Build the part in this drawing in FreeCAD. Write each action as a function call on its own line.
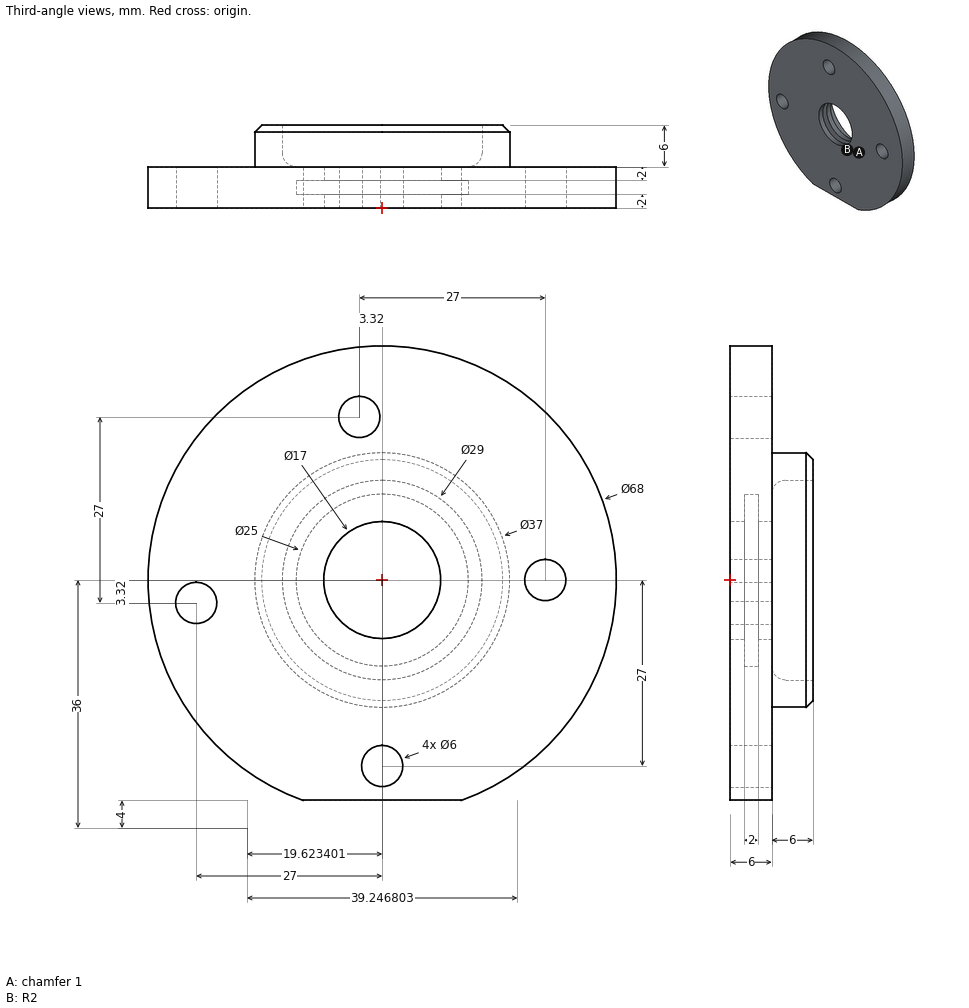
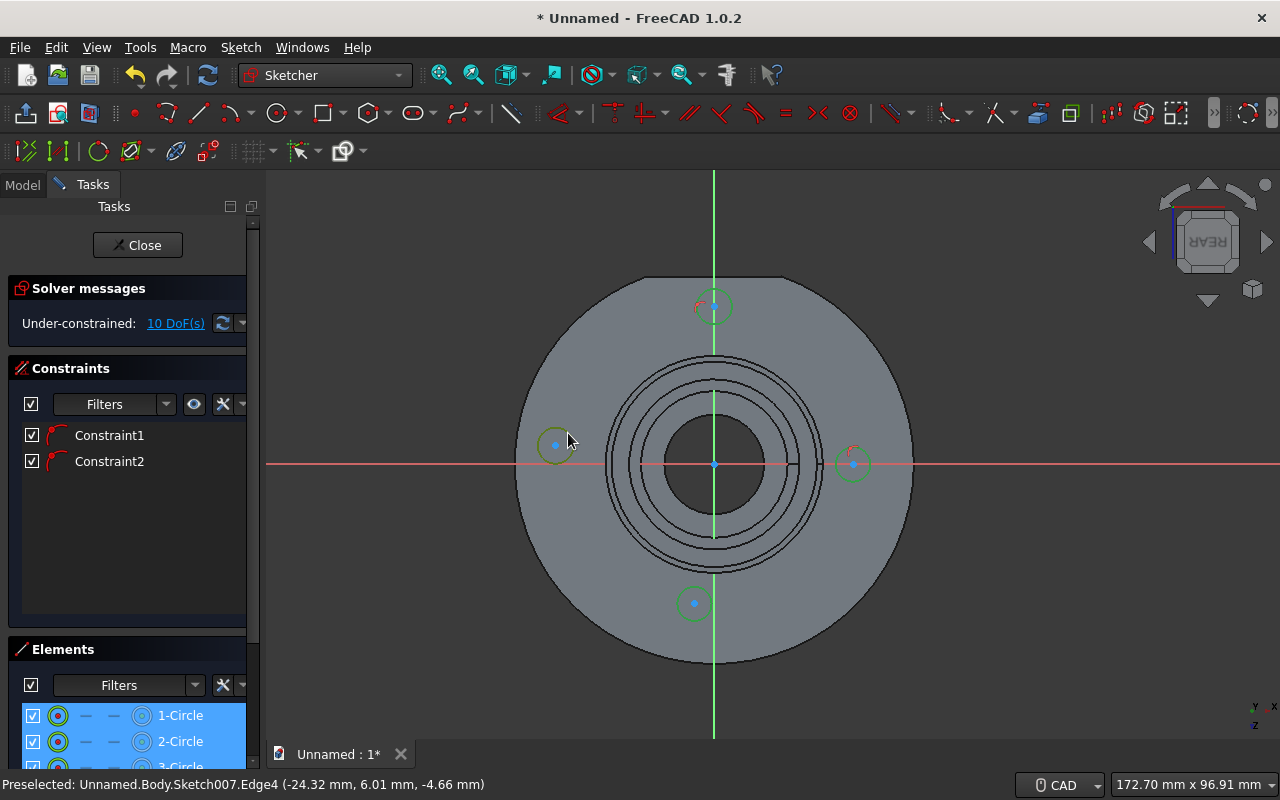
click(786, 114)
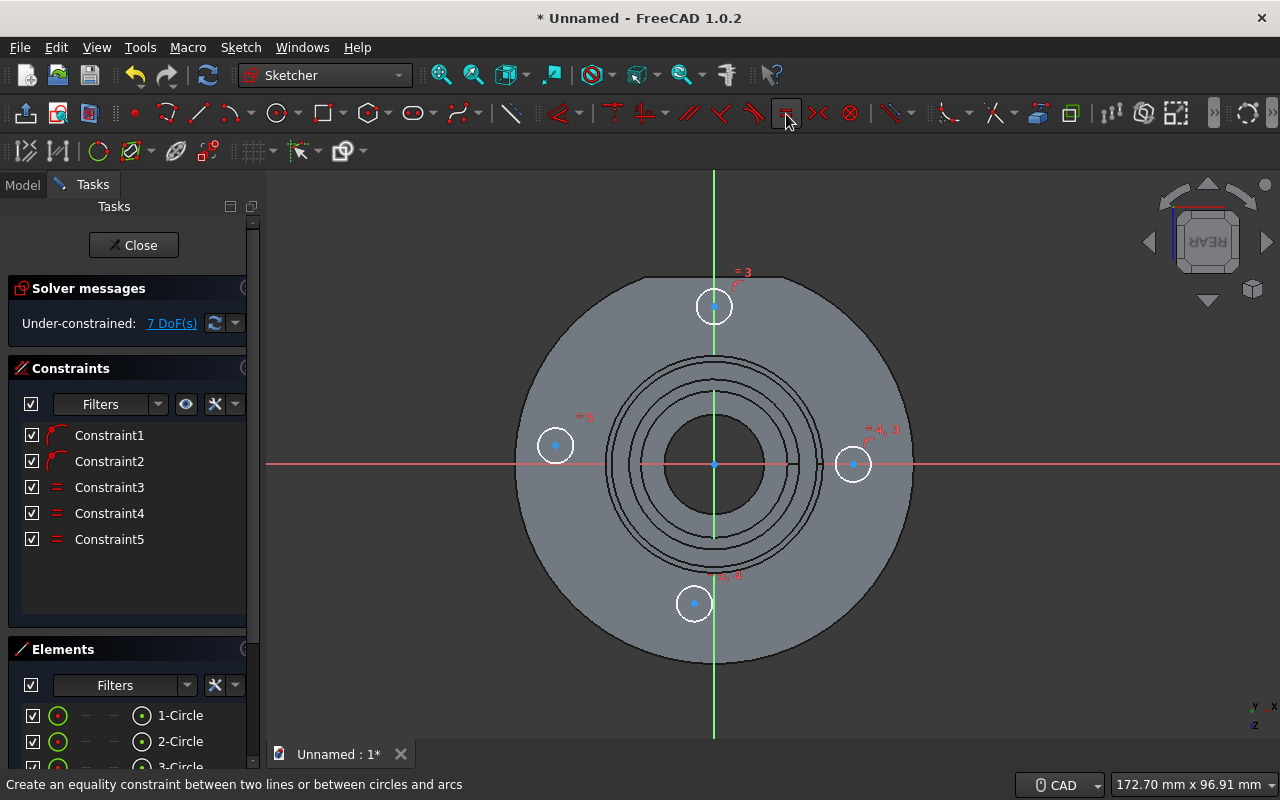
click(558, 114)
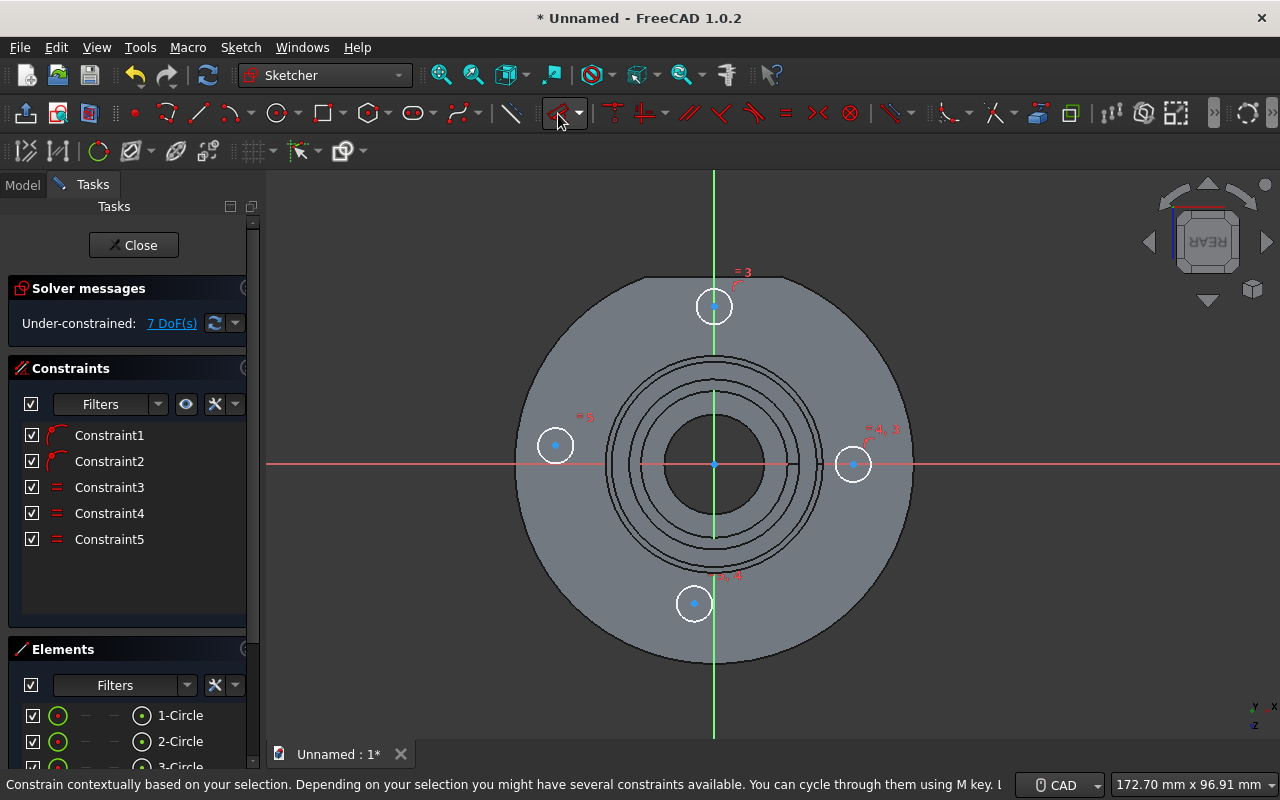
click(727, 294)
click(750, 271)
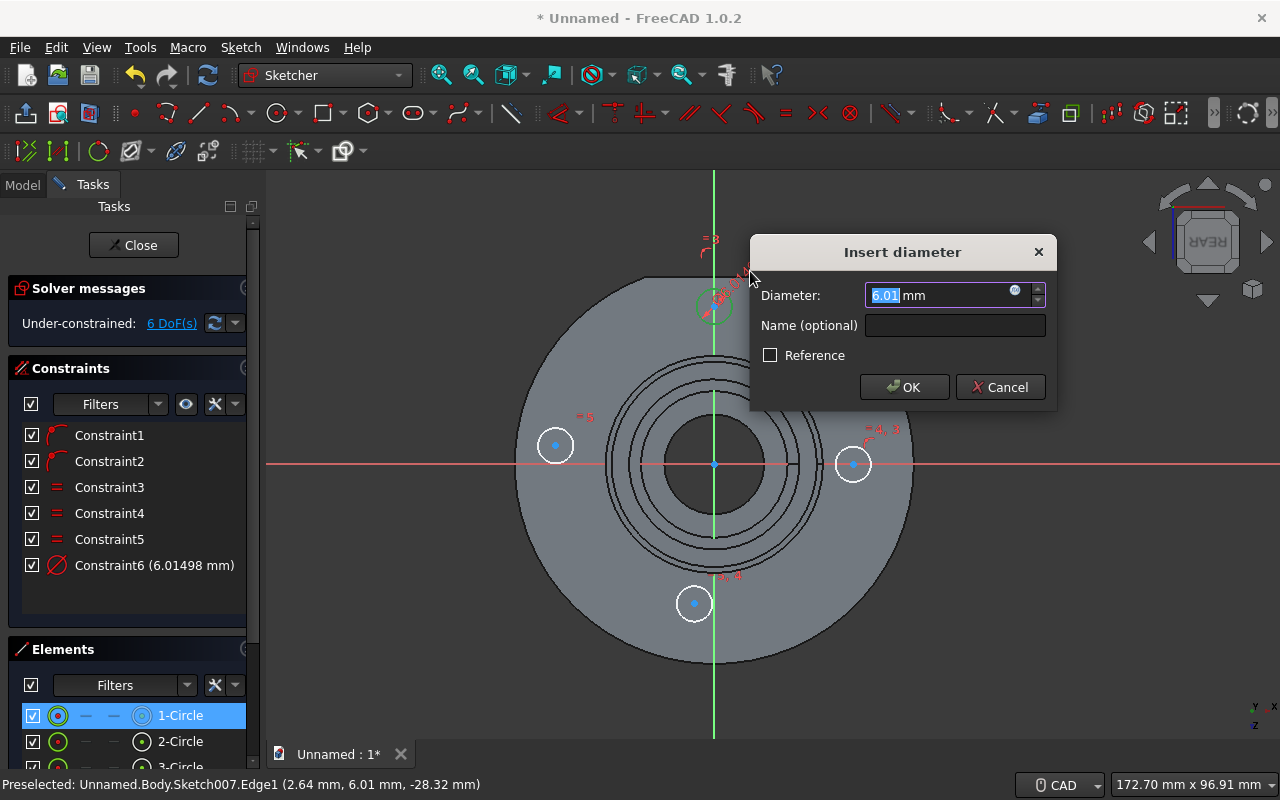
text(6)
key(Return)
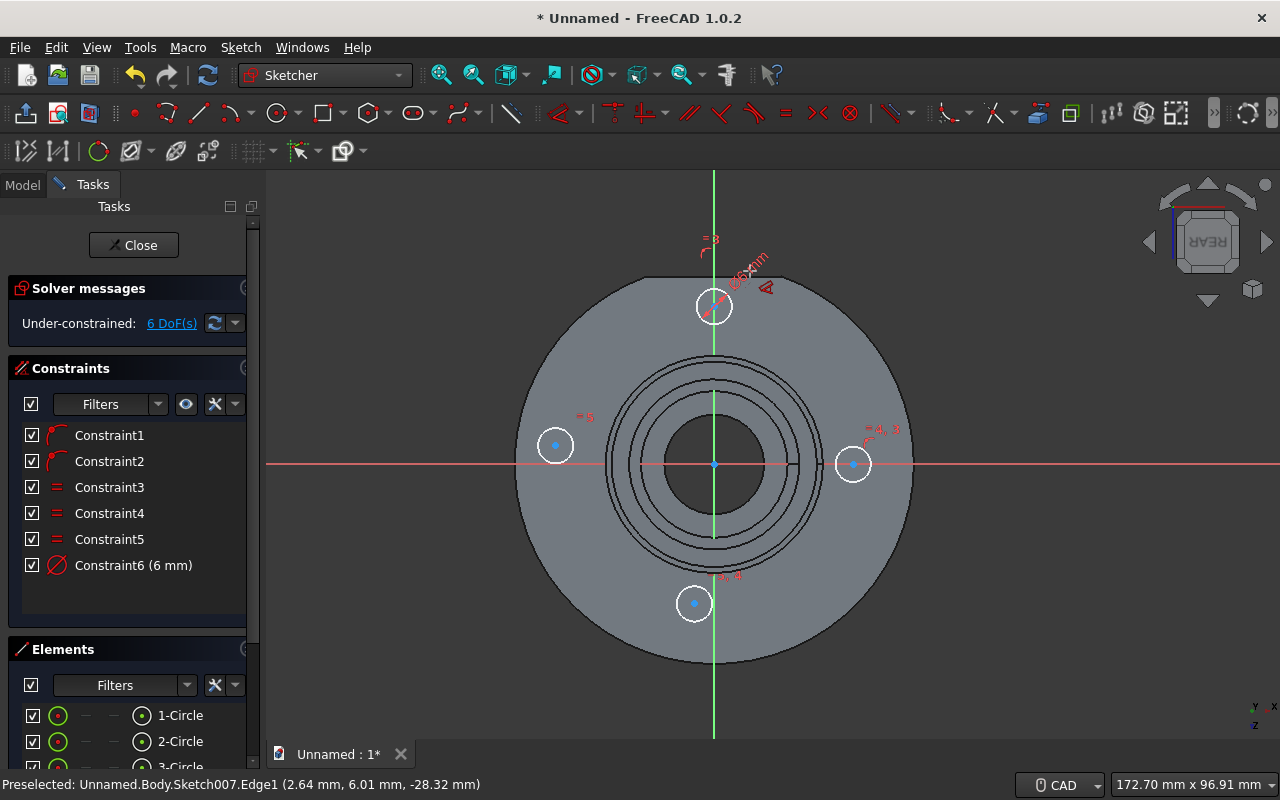
click(714, 307)
click(748, 386)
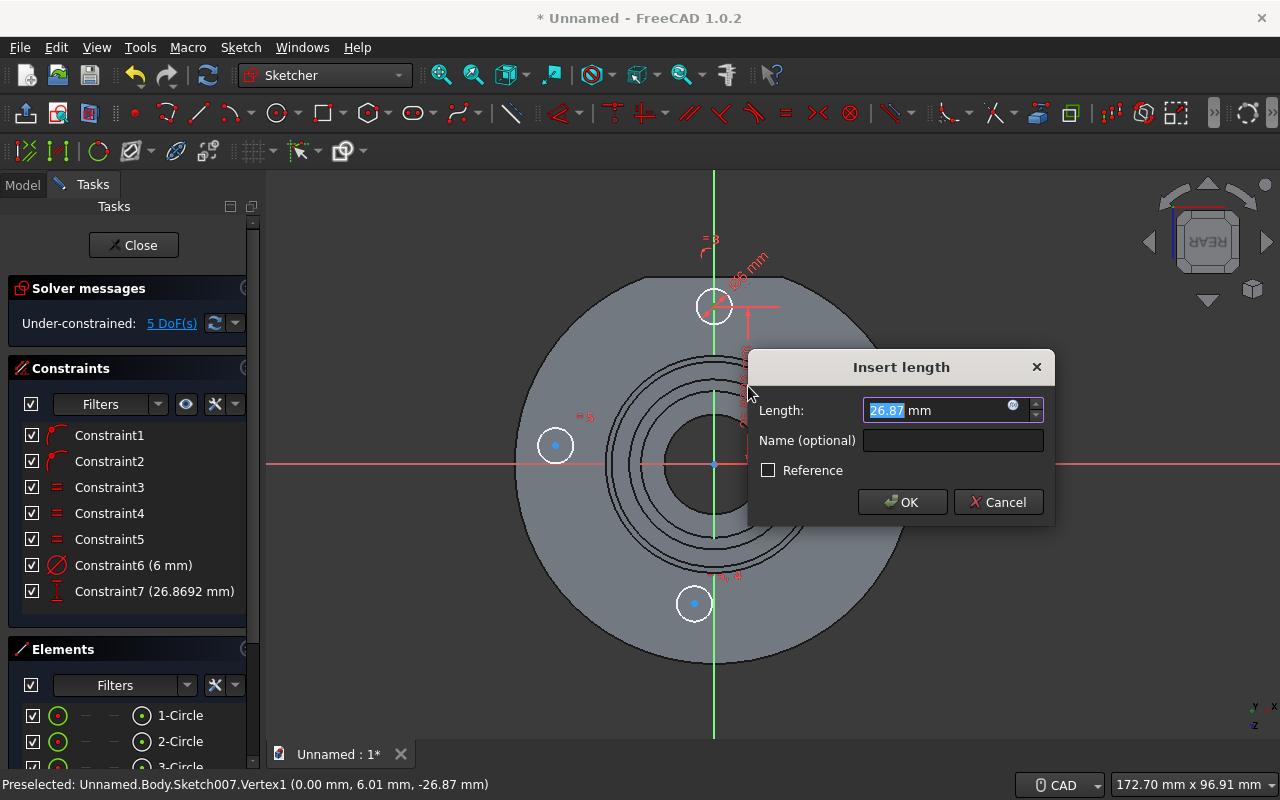
text(27)
key(Return)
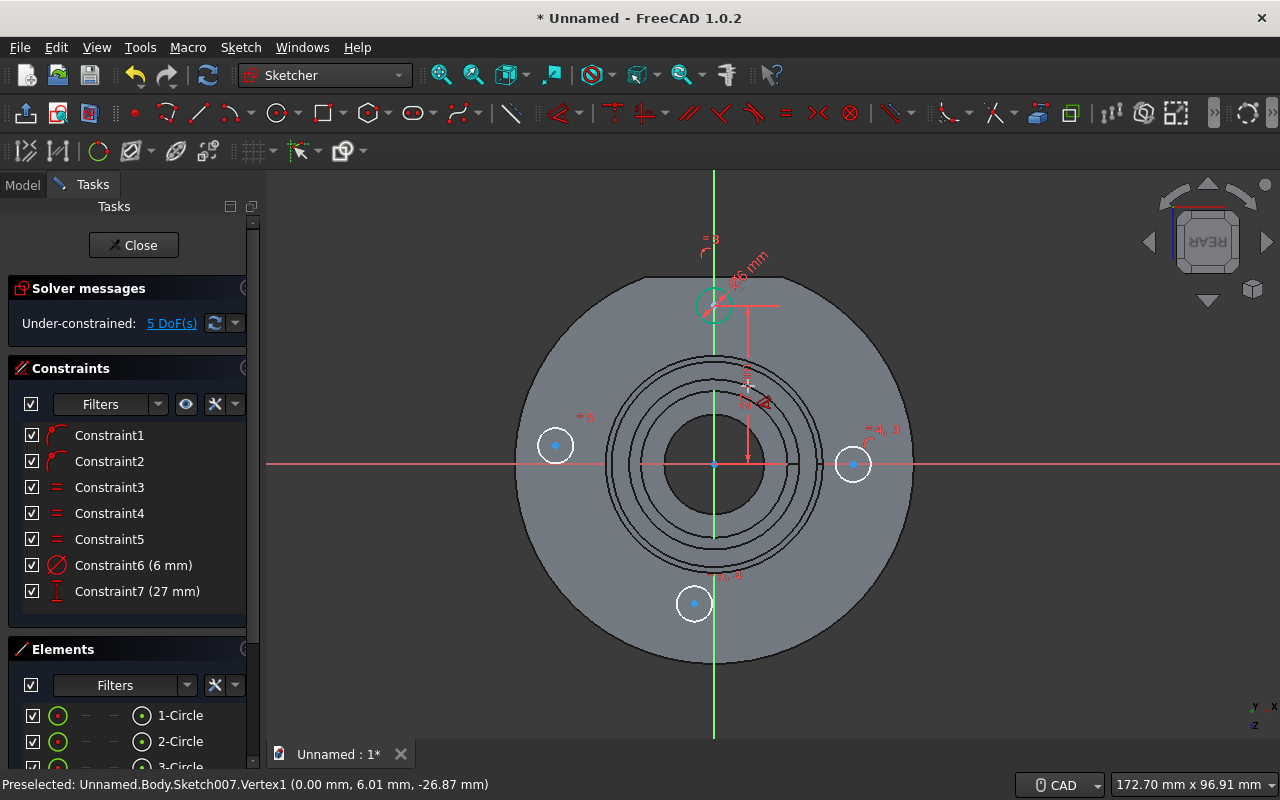
click(556, 446)
click(635, 498)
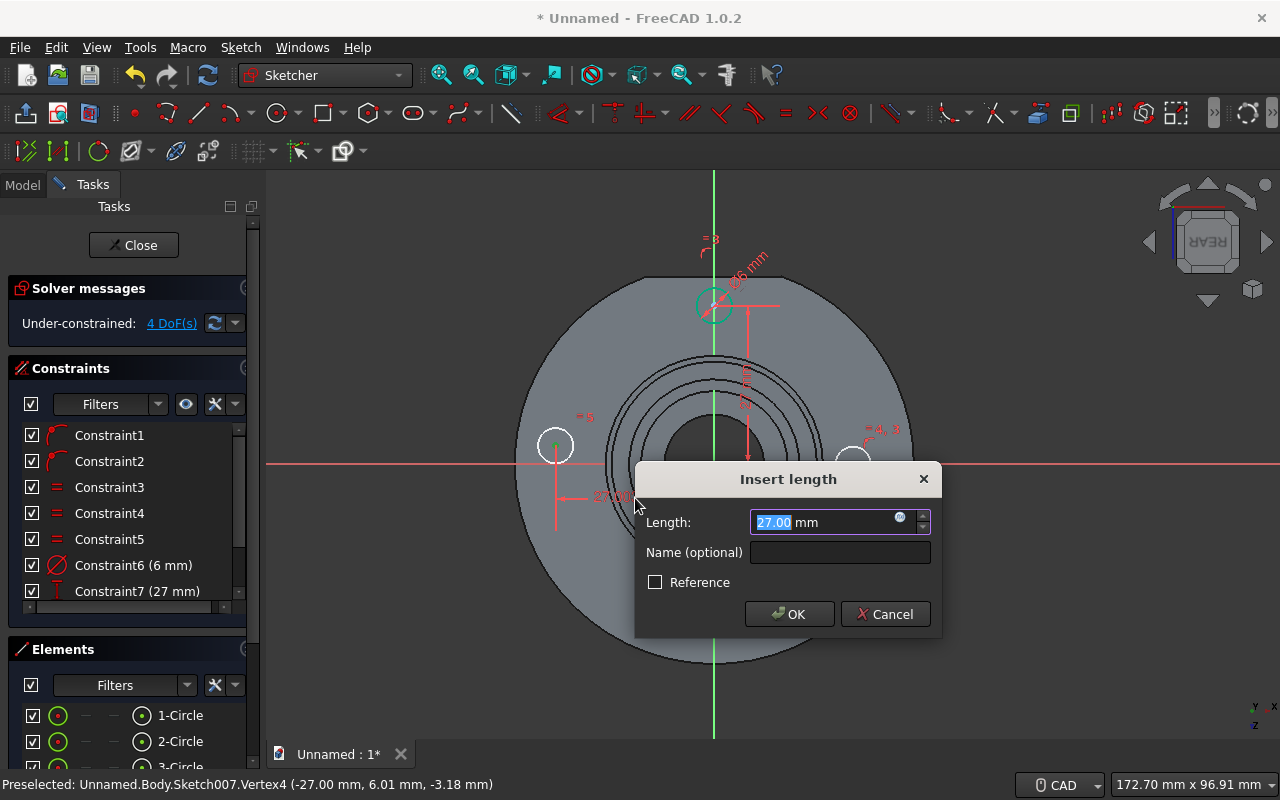
text(27)
key(Return)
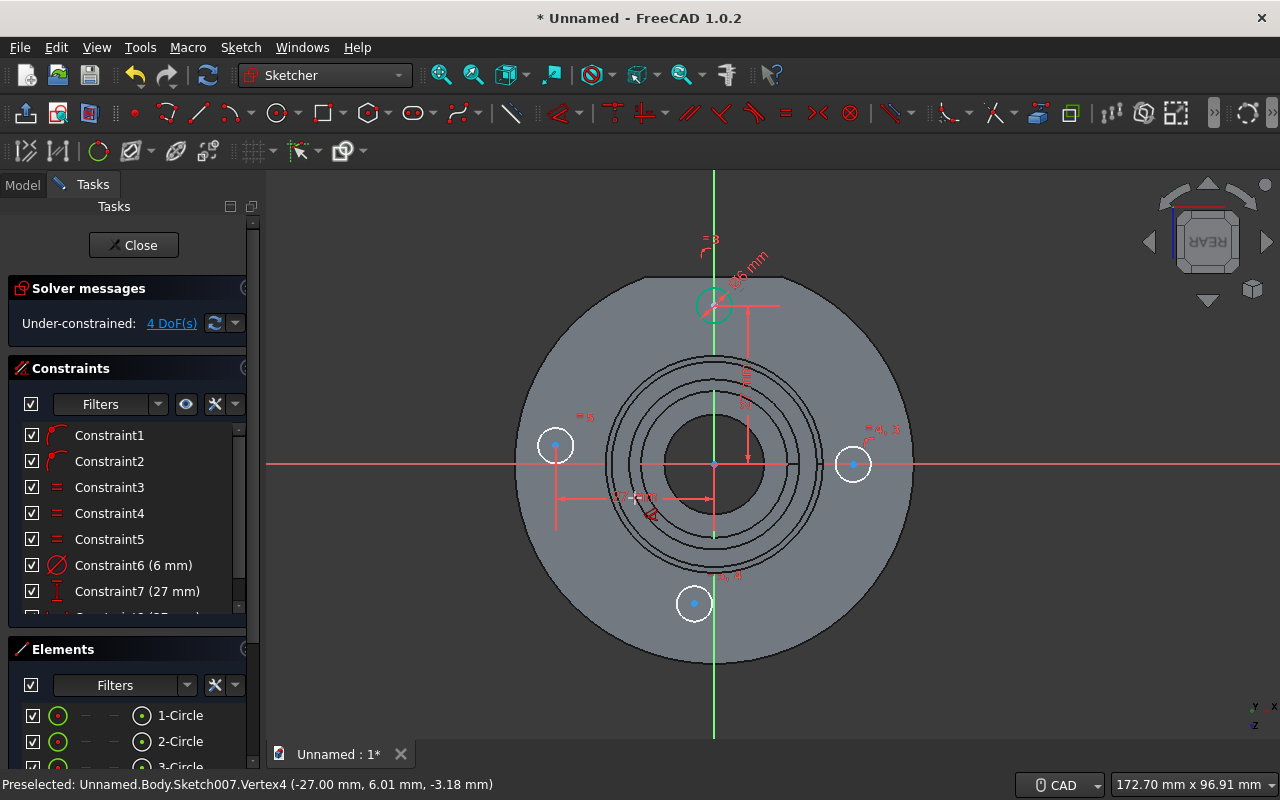
click(853, 464)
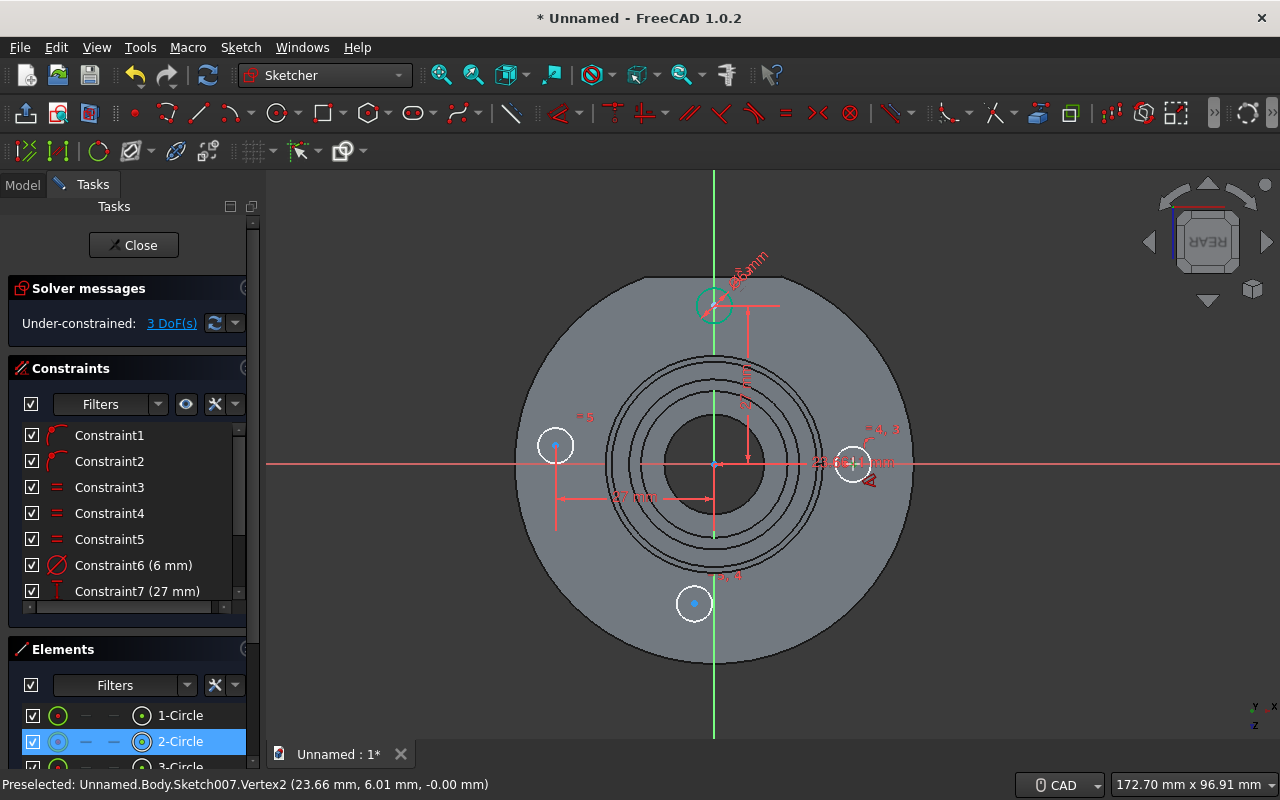
click(694, 604)
click(774, 638)